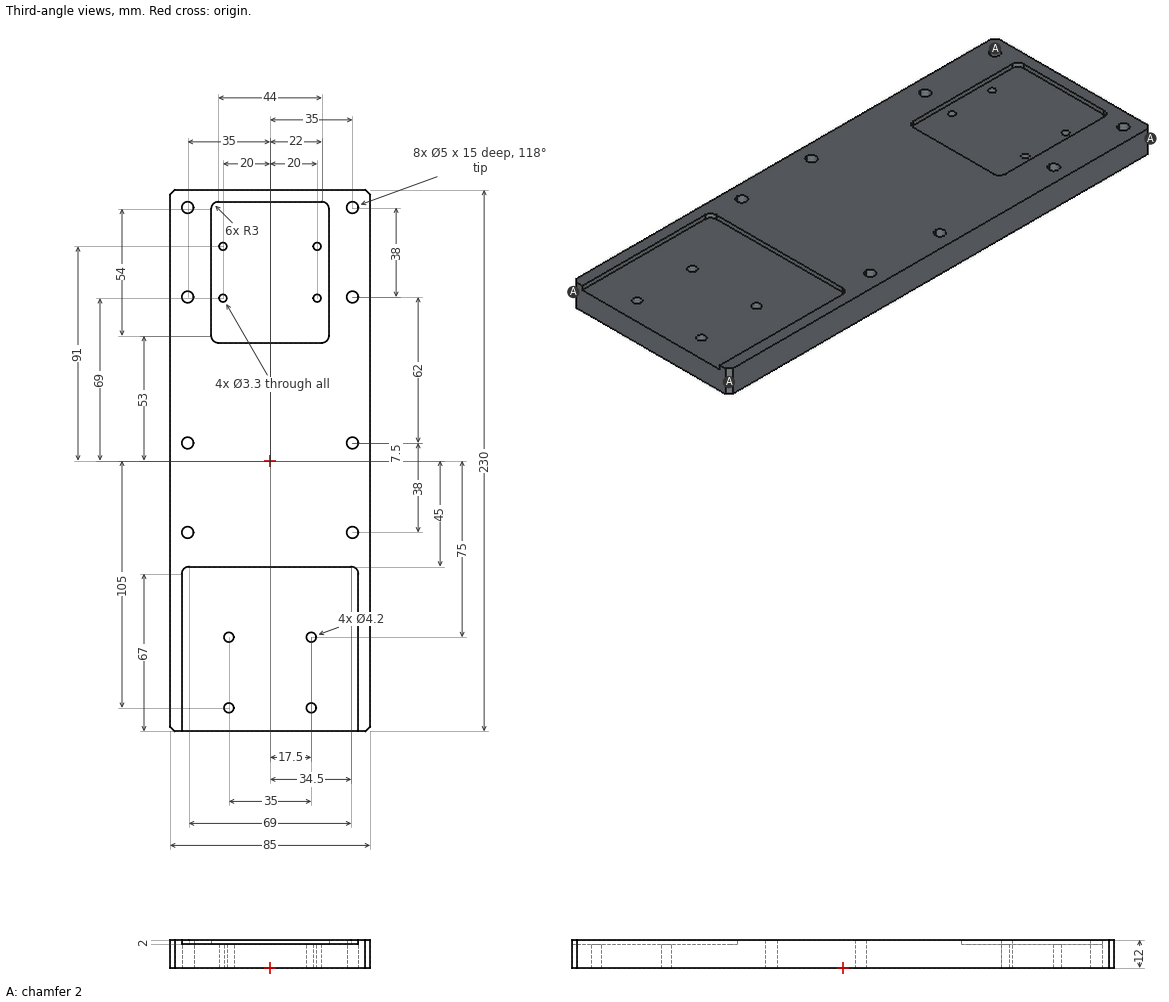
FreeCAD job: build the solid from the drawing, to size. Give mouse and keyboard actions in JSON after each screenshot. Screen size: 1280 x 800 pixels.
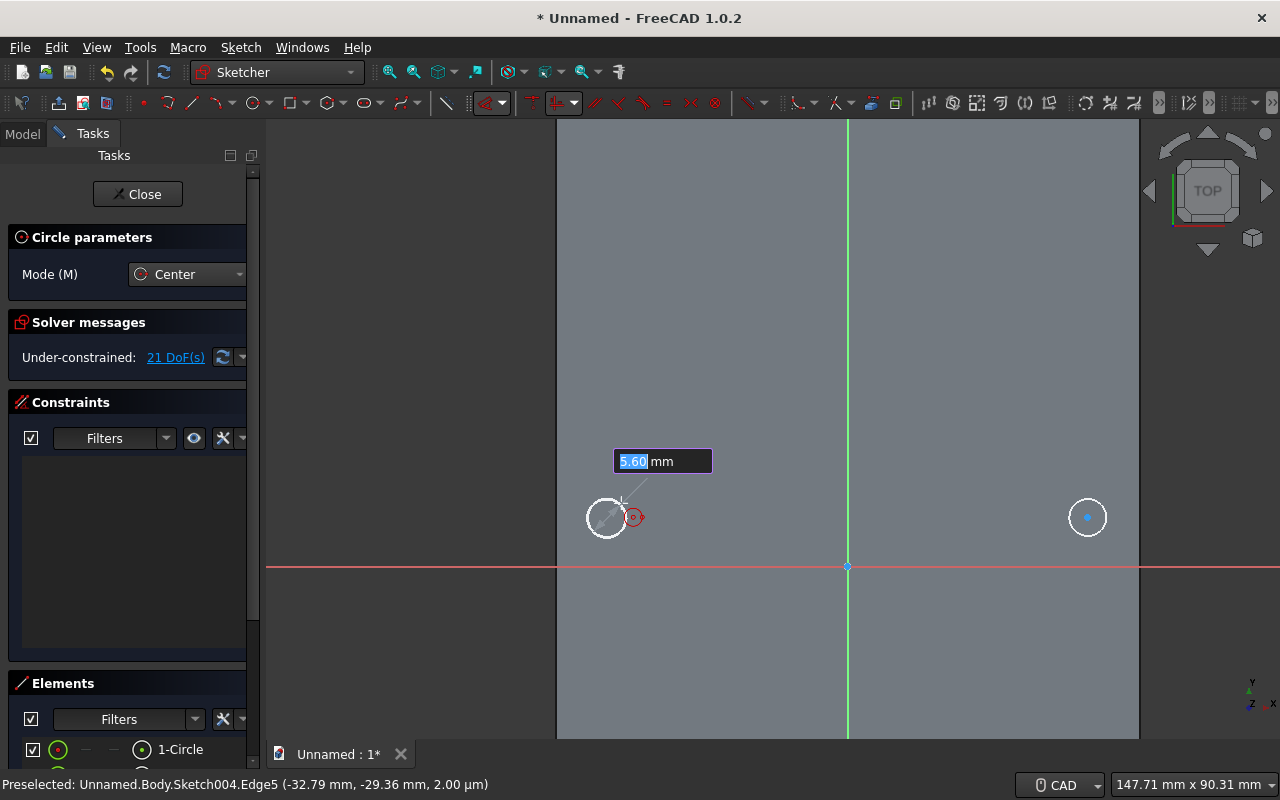
{"action": "left_click", "coordinate": [620, 503]}
{"action": "key", "text": "Escape"}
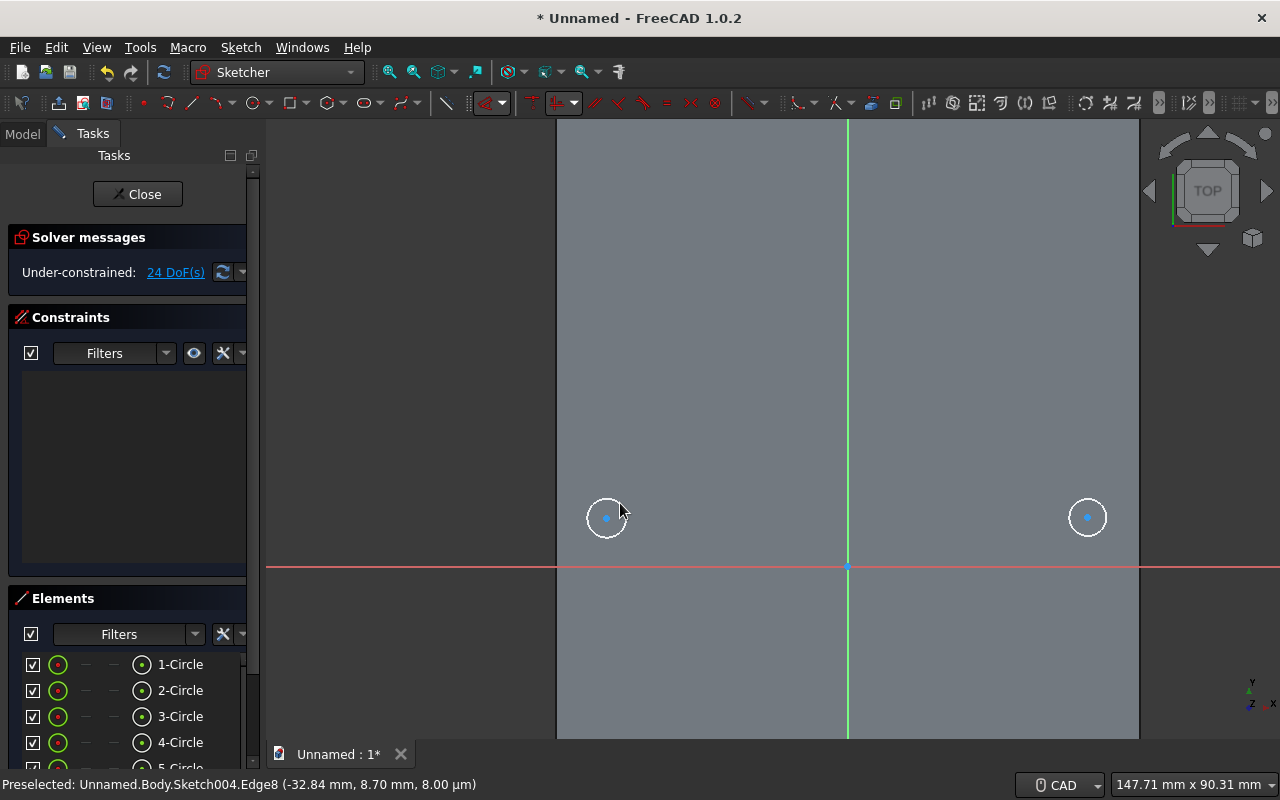
{"action": "scroll", "coordinate": [621, 503], "scroll_direction": "down", "scroll_amount": 5}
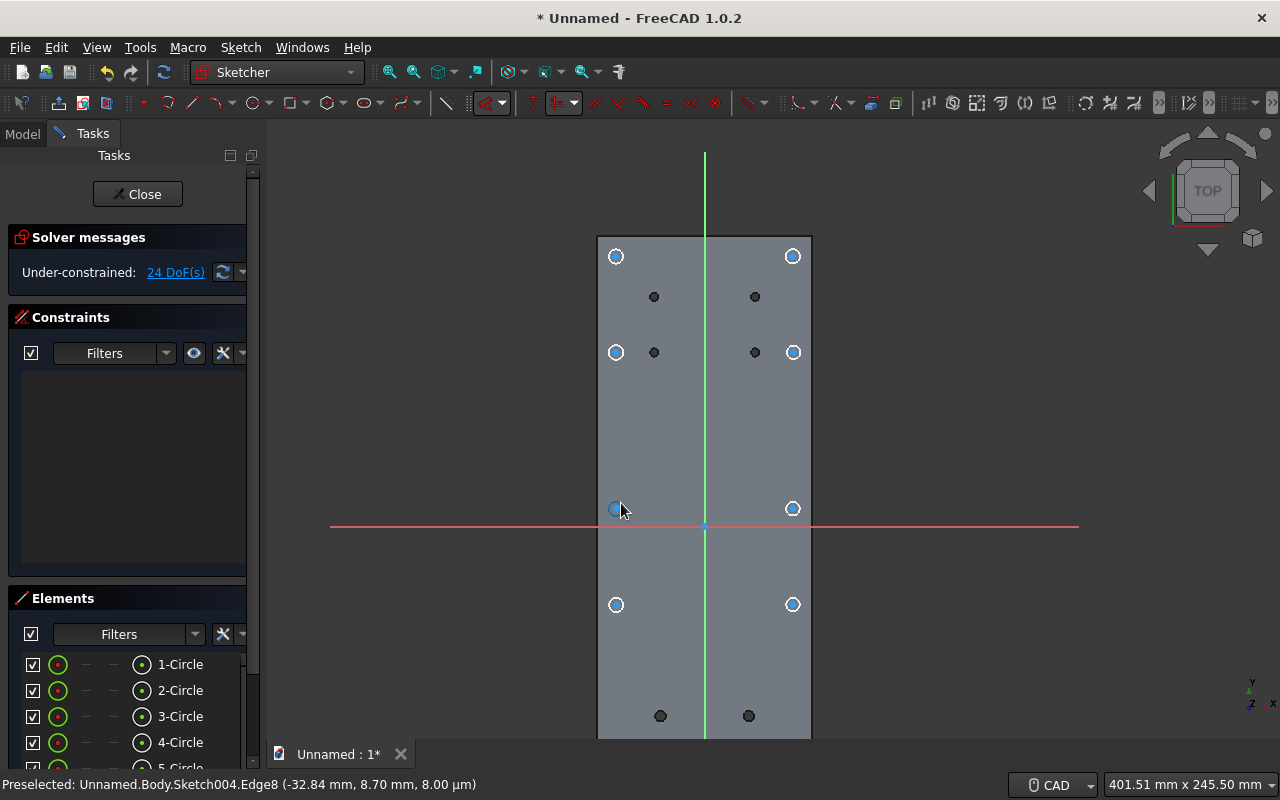
{"action": "scroll", "coordinate": [798, 251], "scroll_direction": "up", "scroll_amount": 4}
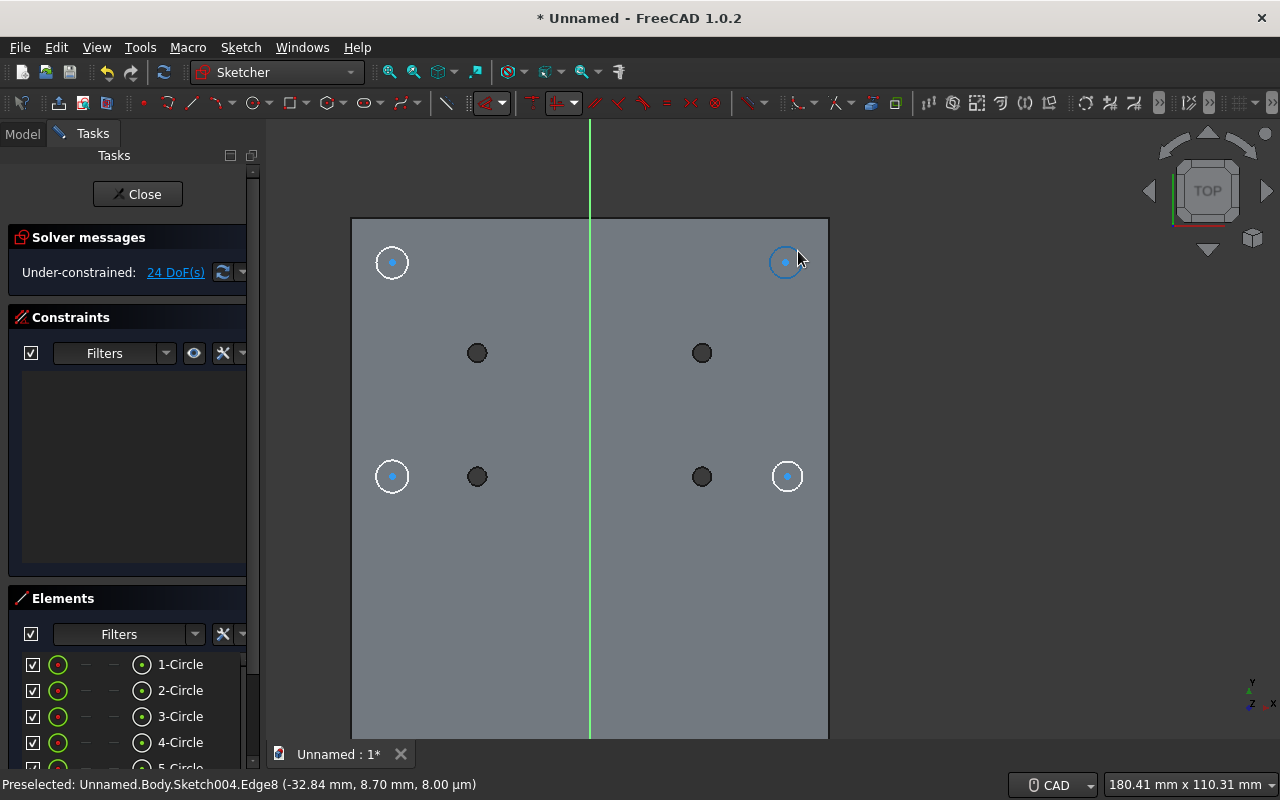
{"action": "left_click", "coordinate": [797, 251]}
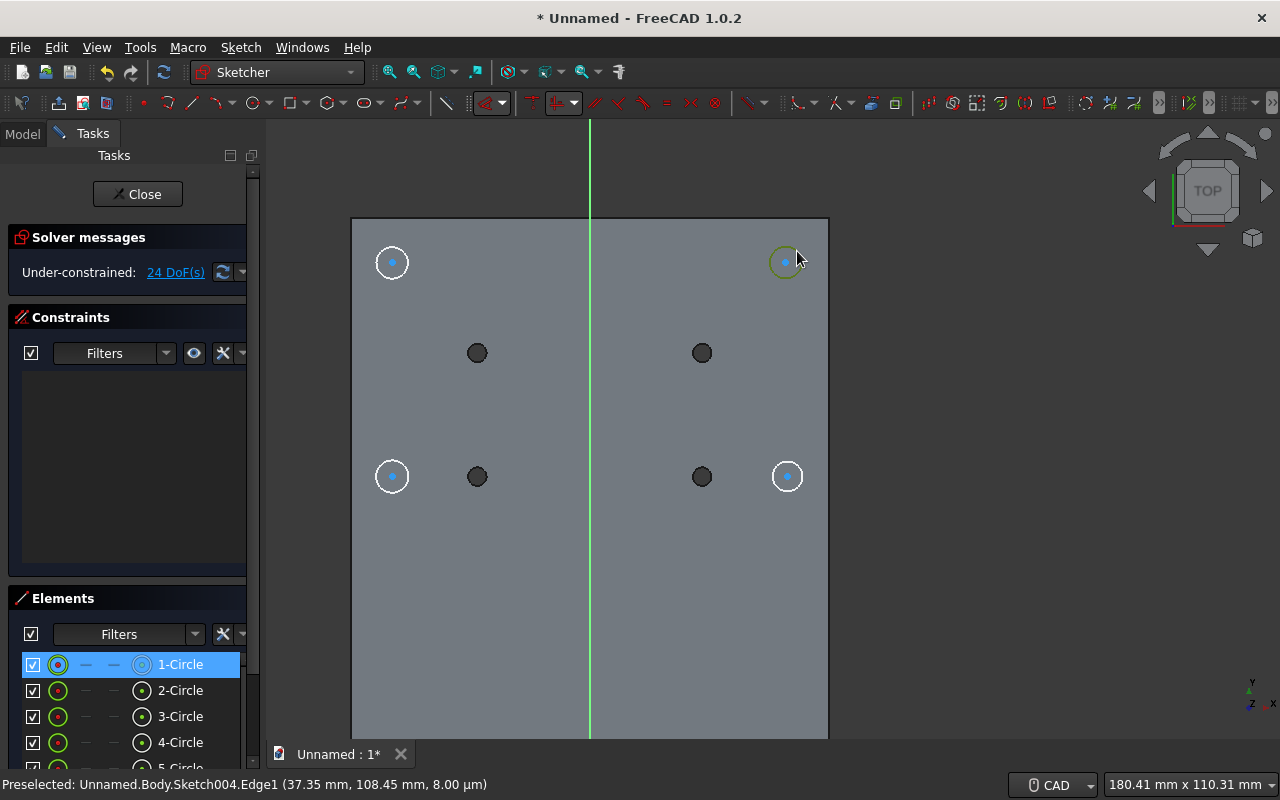
{"action": "left_click", "coordinate": [798, 466]}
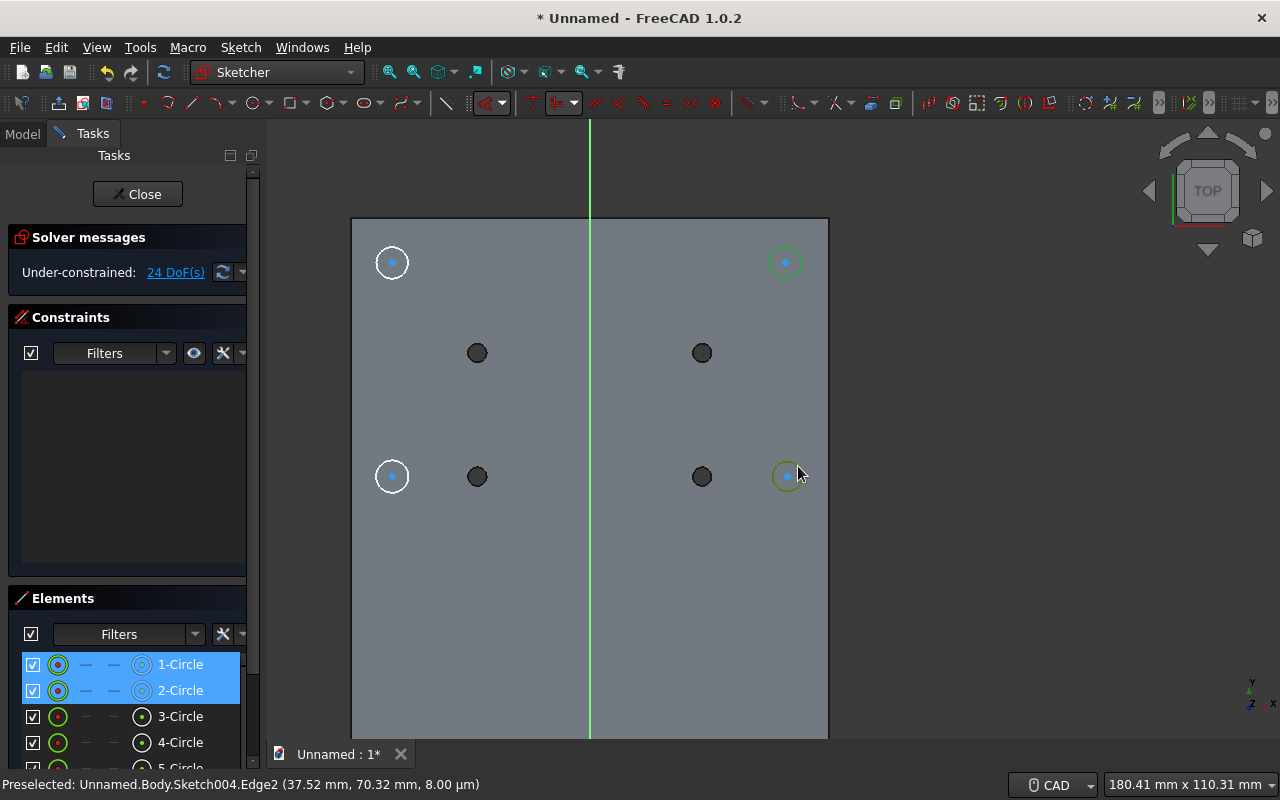
{"action": "left_click", "coordinate": [404, 465]}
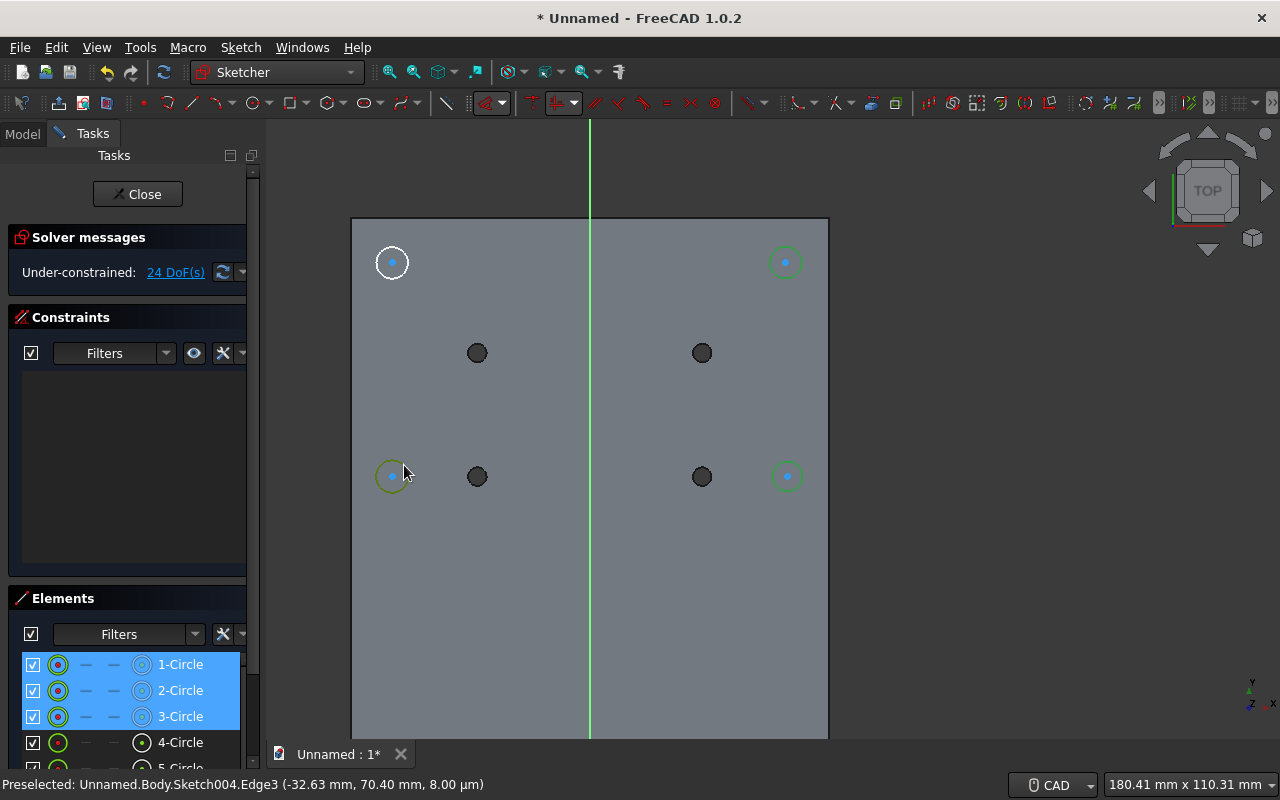
{"action": "left_click", "coordinate": [403, 252]}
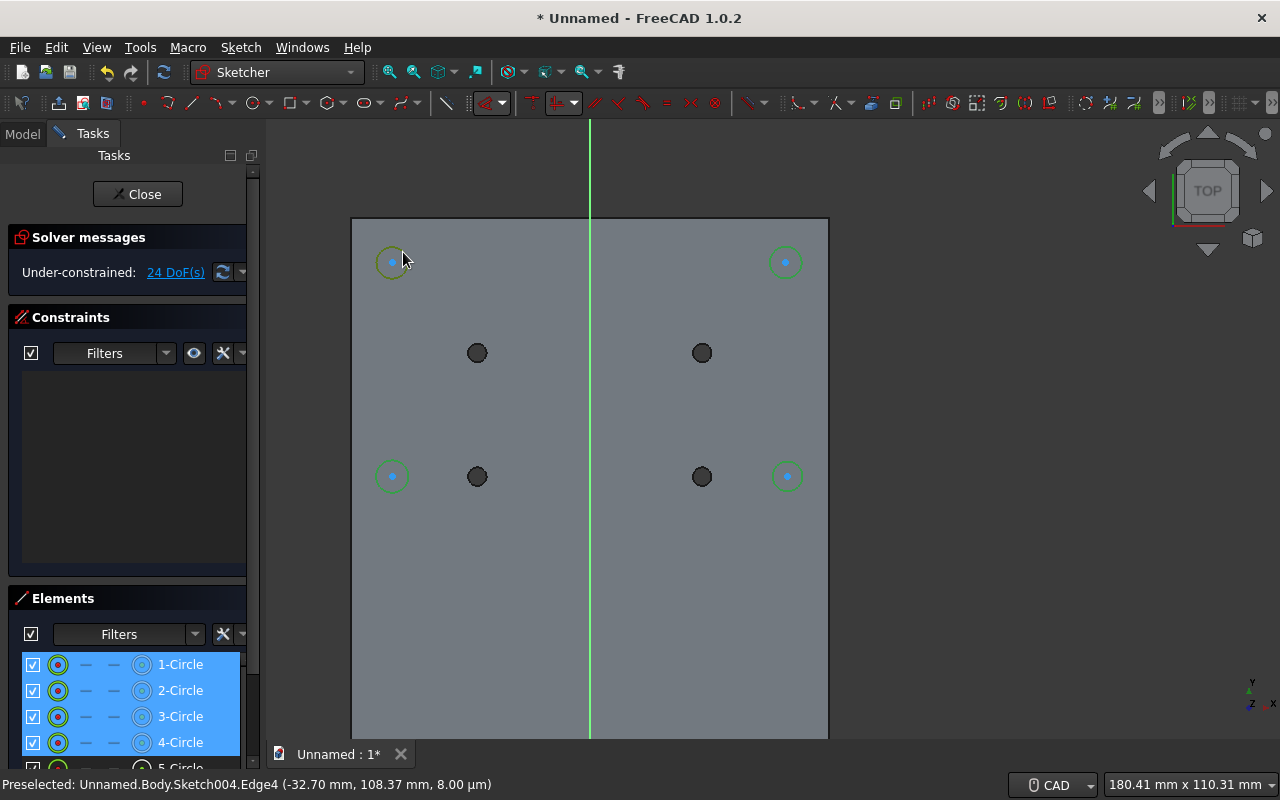
{"action": "scroll", "coordinate": [798, 250], "scroll_direction": "down", "scroll_amount": 4}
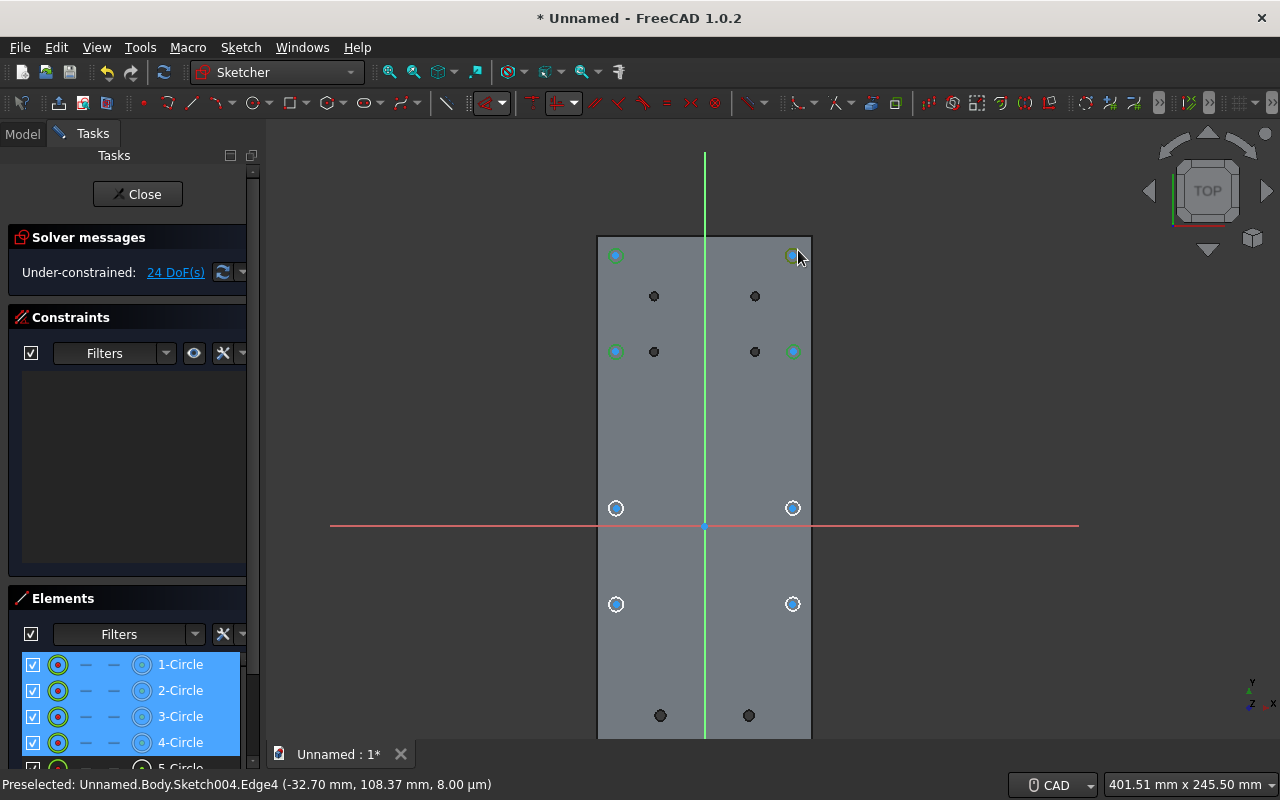
{"action": "scroll", "coordinate": [798, 503], "scroll_direction": "up", "scroll_amount": 4}